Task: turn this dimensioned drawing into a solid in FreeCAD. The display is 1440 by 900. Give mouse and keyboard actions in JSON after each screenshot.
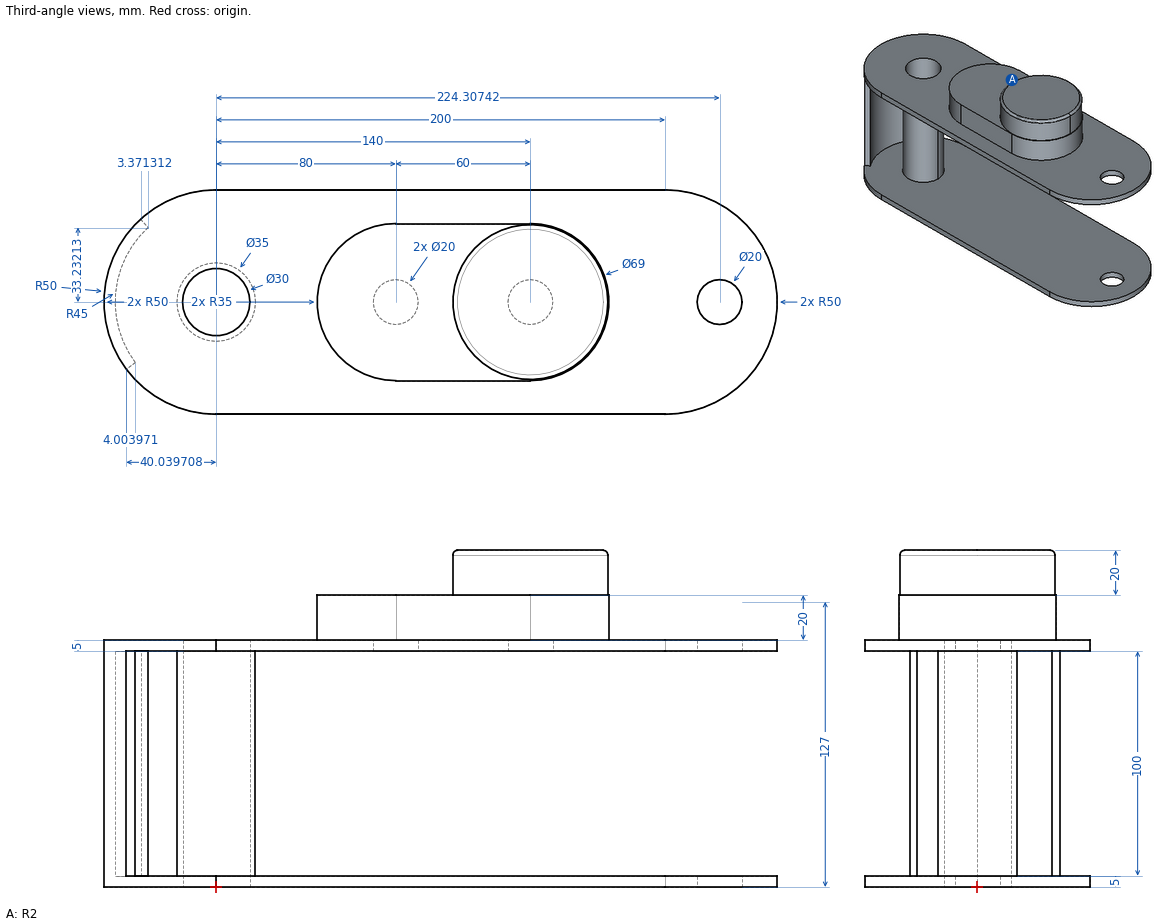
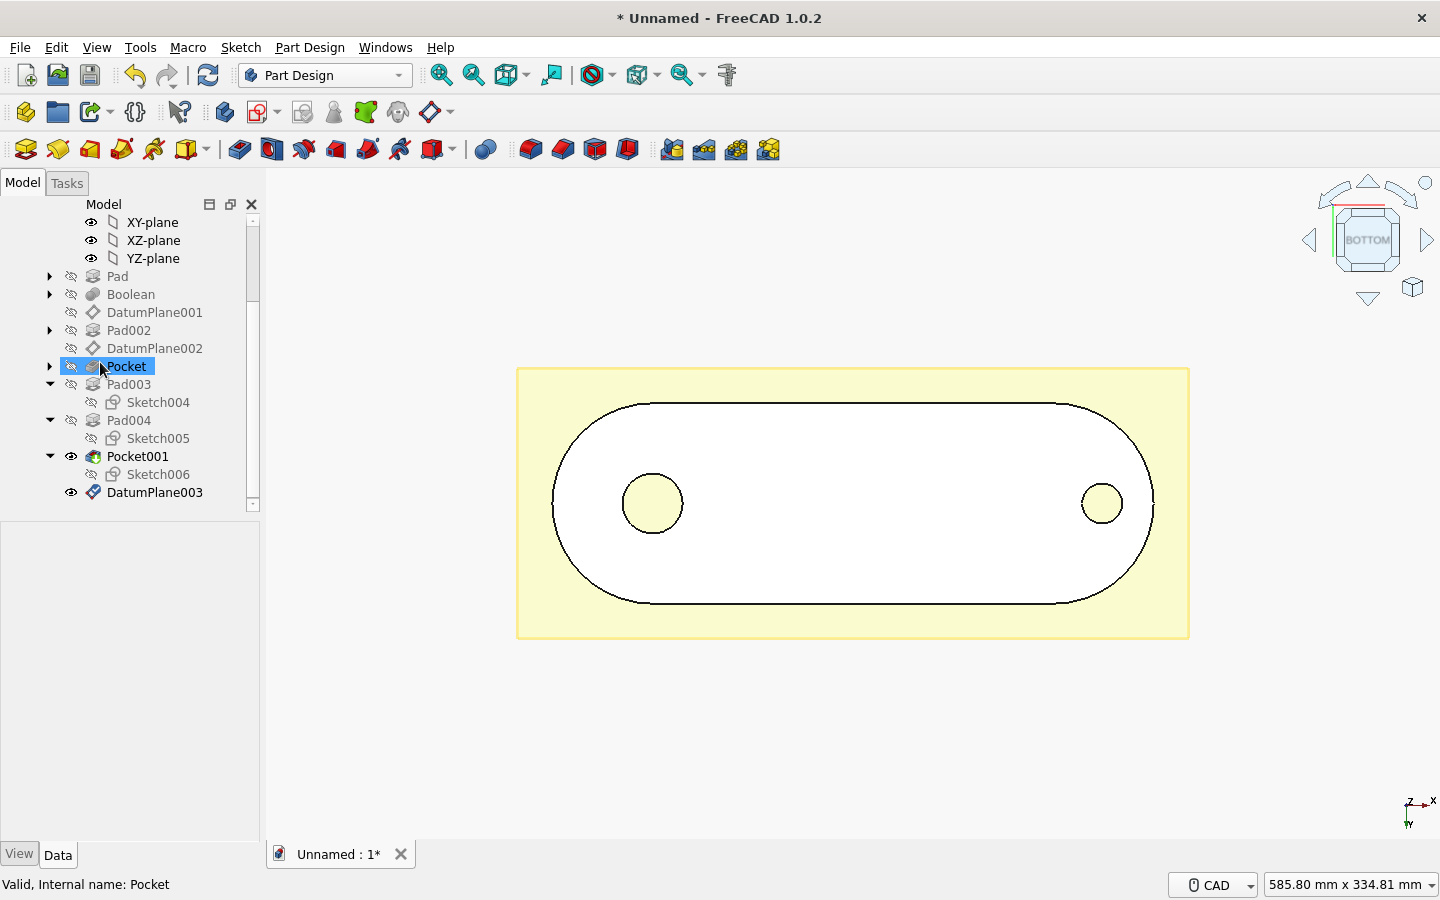
{"action": "left_click", "coordinate": [116, 492]}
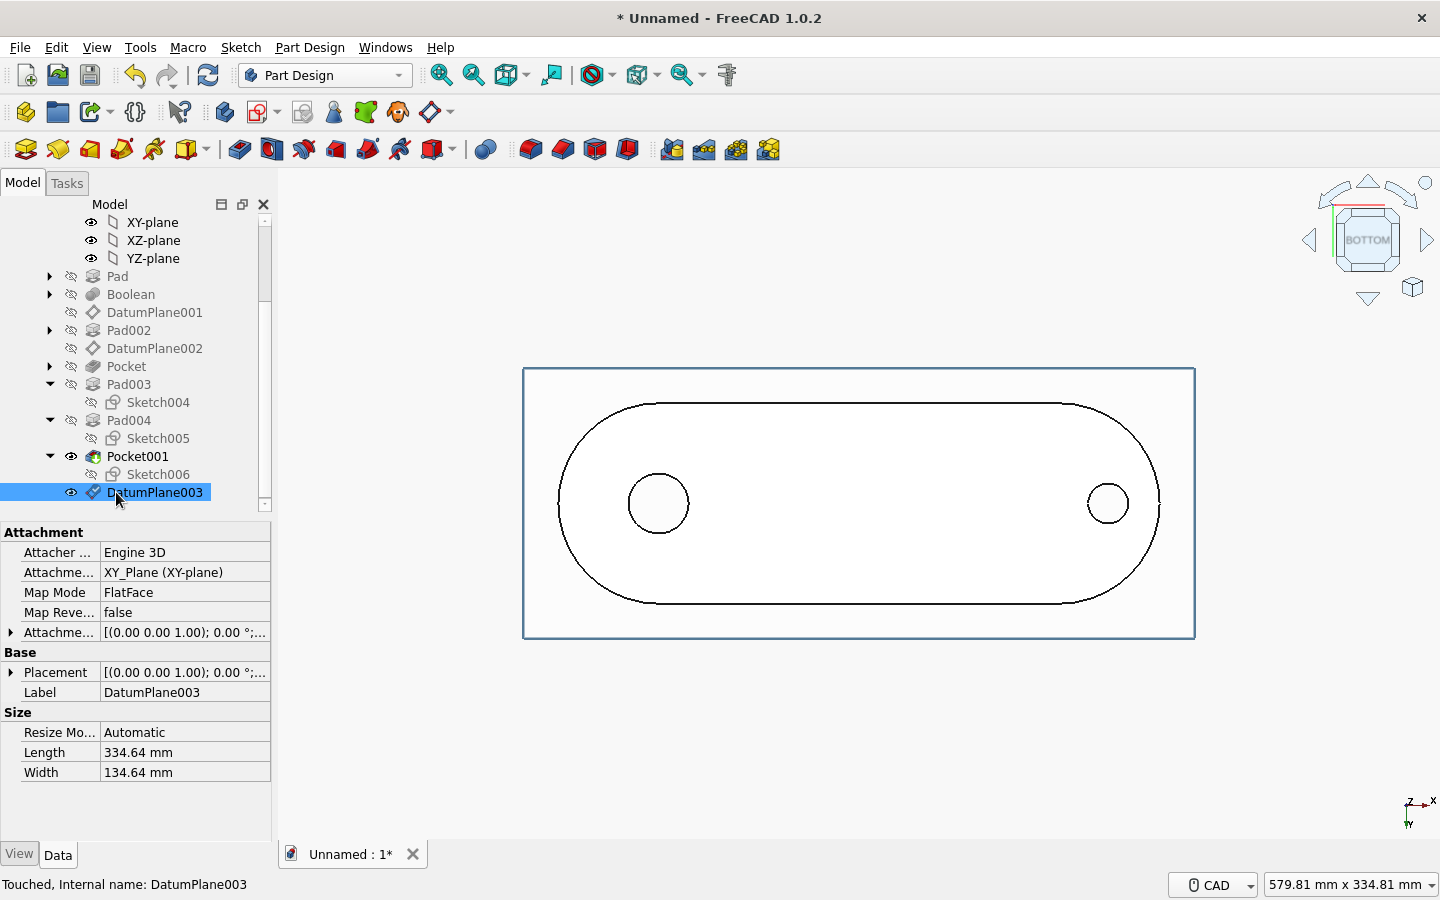
{"action": "left_click", "coordinate": [258, 112]}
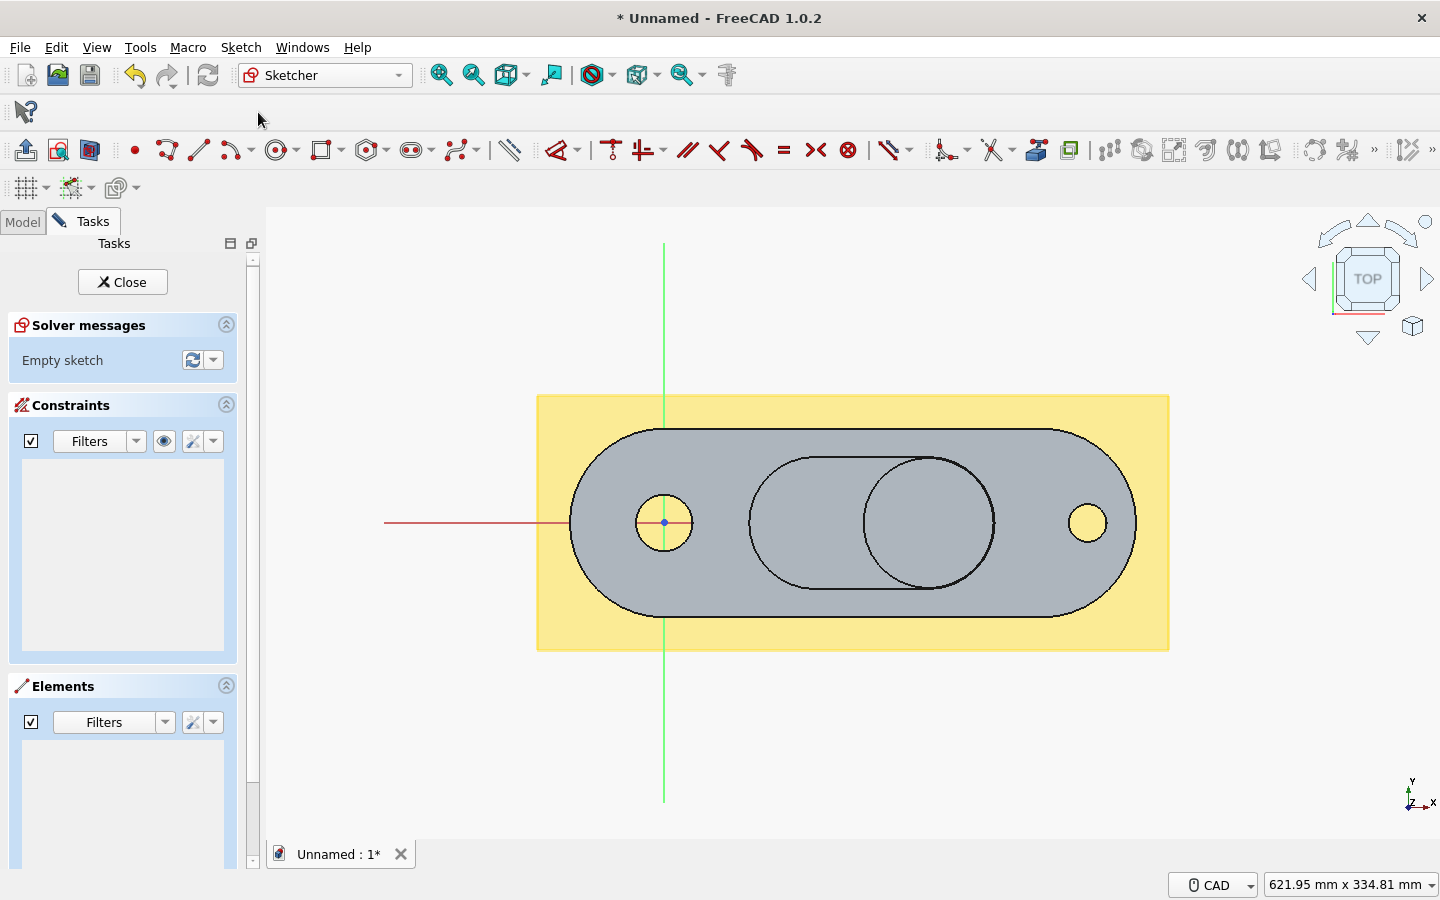
{"action": "left_click", "coordinate": [90, 150]}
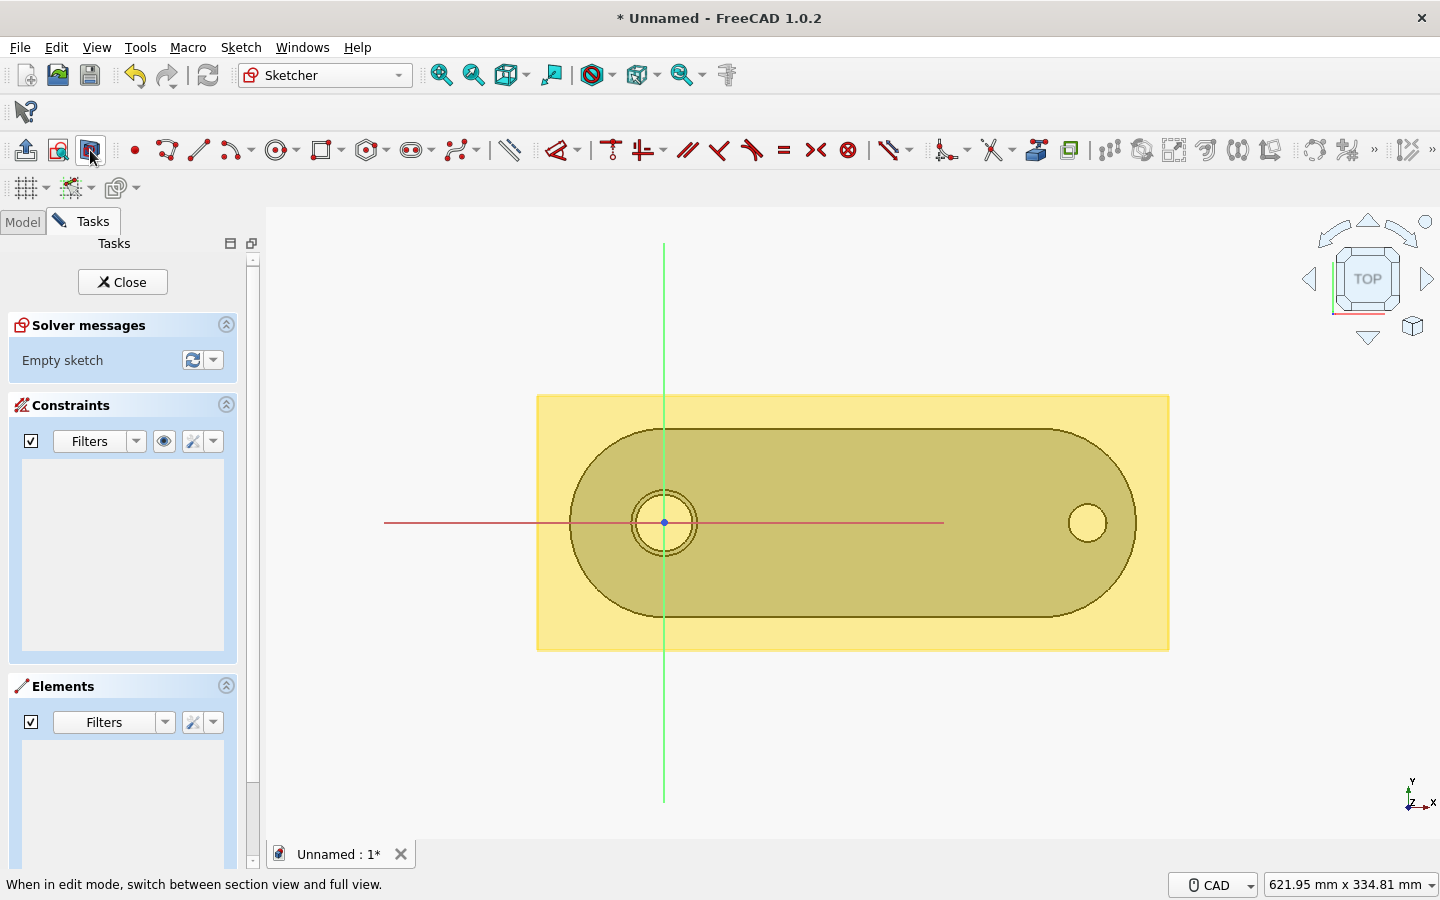
{"action": "scroll", "coordinate": [545, 514], "scroll_direction": "up", "scroll_amount": 6}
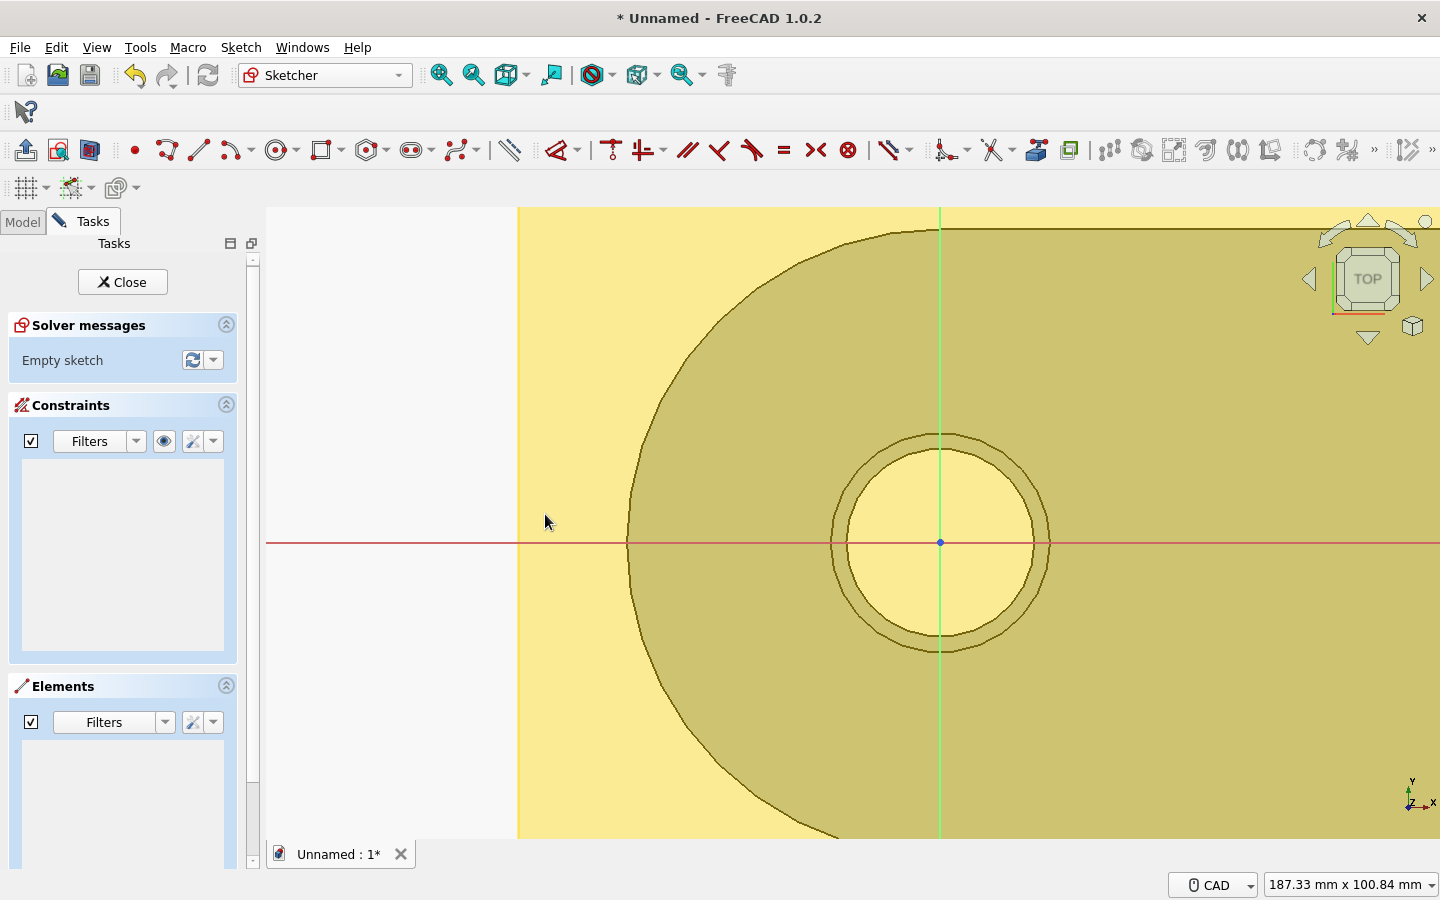
{"action": "left_click", "coordinate": [200, 150]}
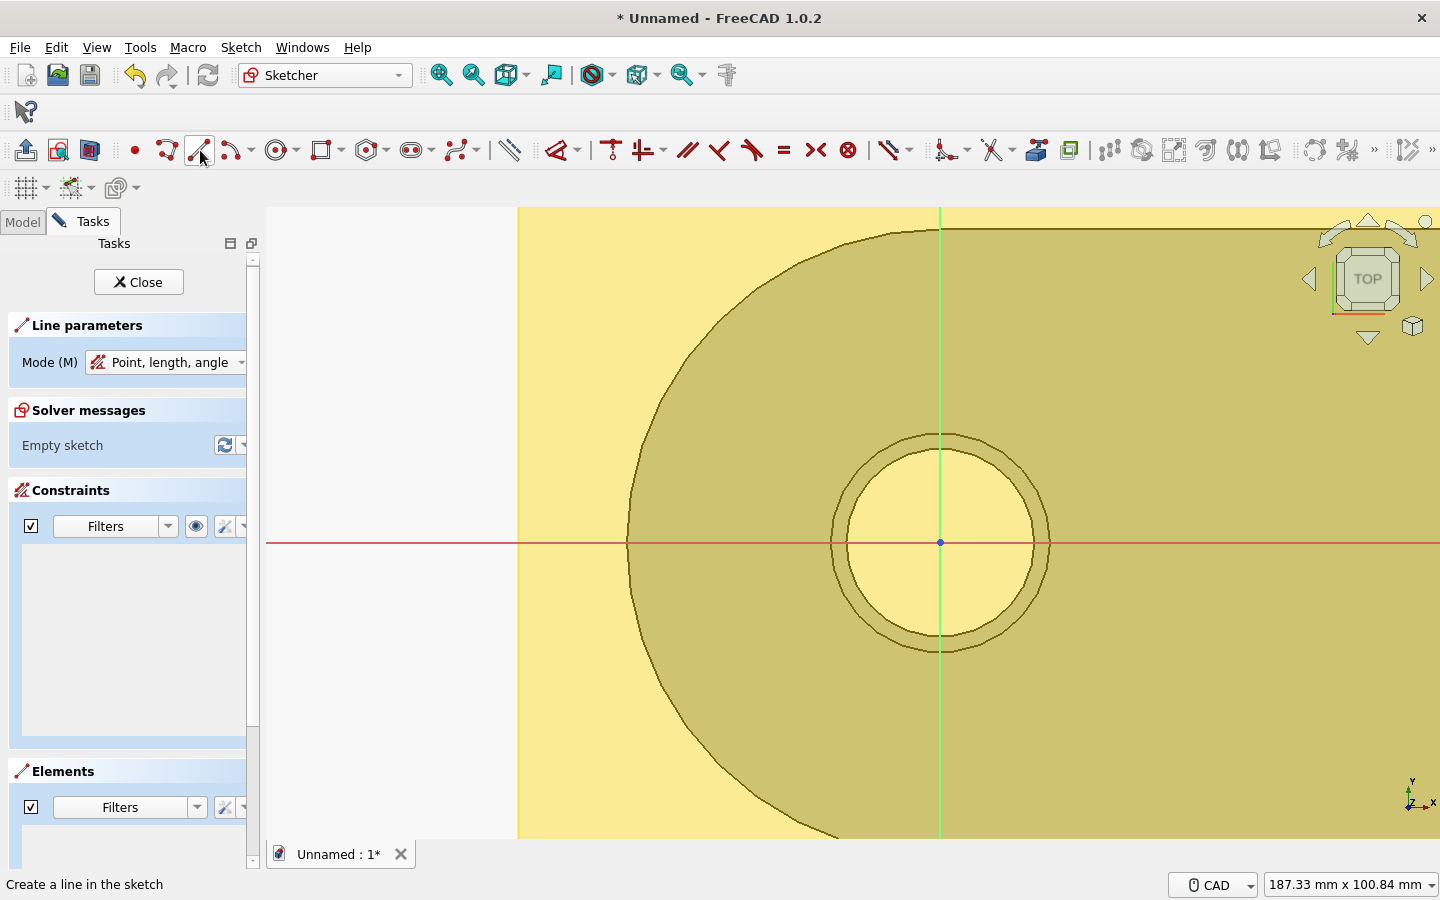
{"action": "left_click", "coordinate": [750, 334]}
{"action": "left_click", "coordinate": [729, 311]}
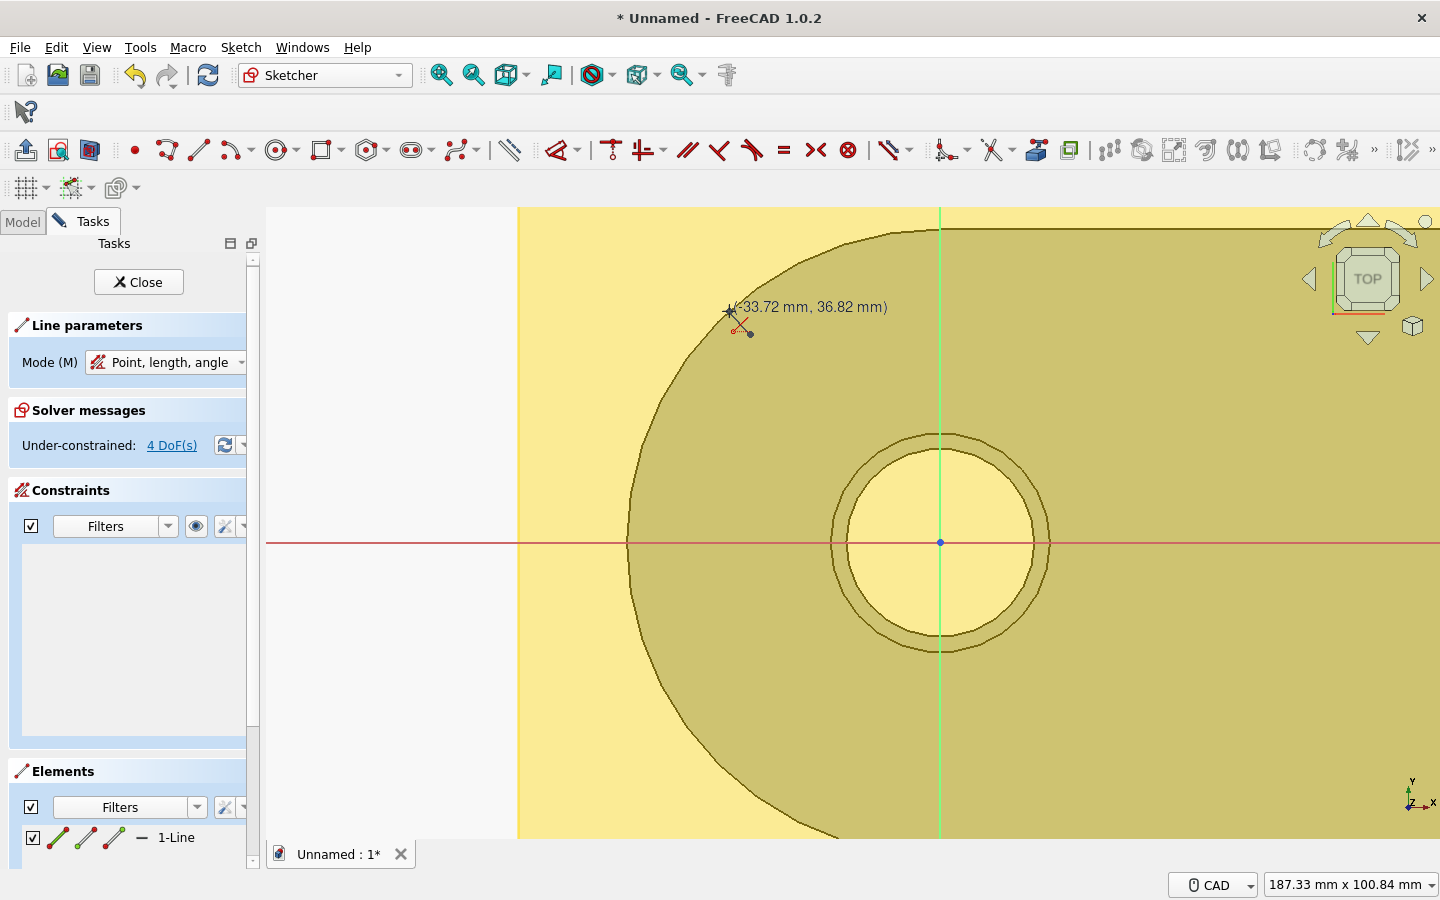
{"action": "left_click", "coordinate": [689, 730]}
{"action": "left_click", "coordinate": [714, 712]}